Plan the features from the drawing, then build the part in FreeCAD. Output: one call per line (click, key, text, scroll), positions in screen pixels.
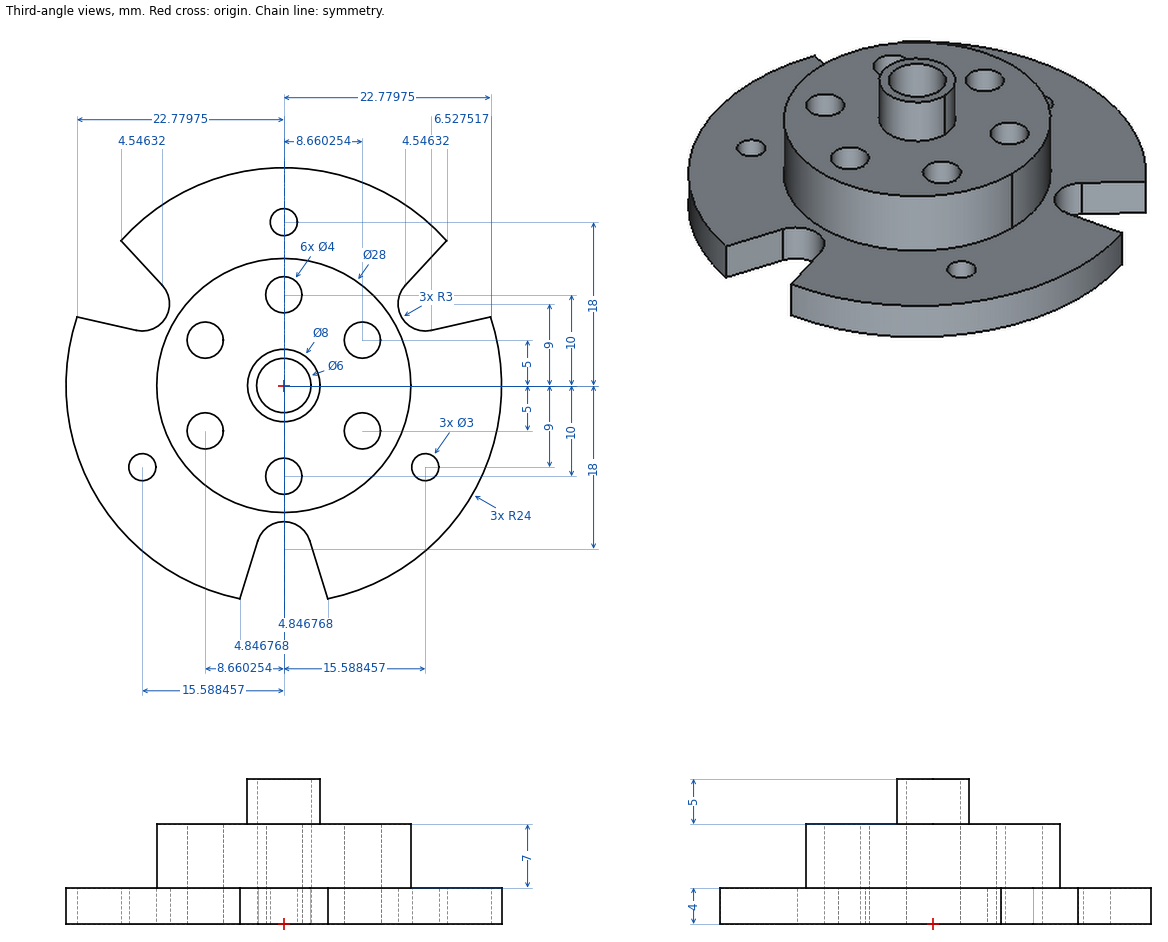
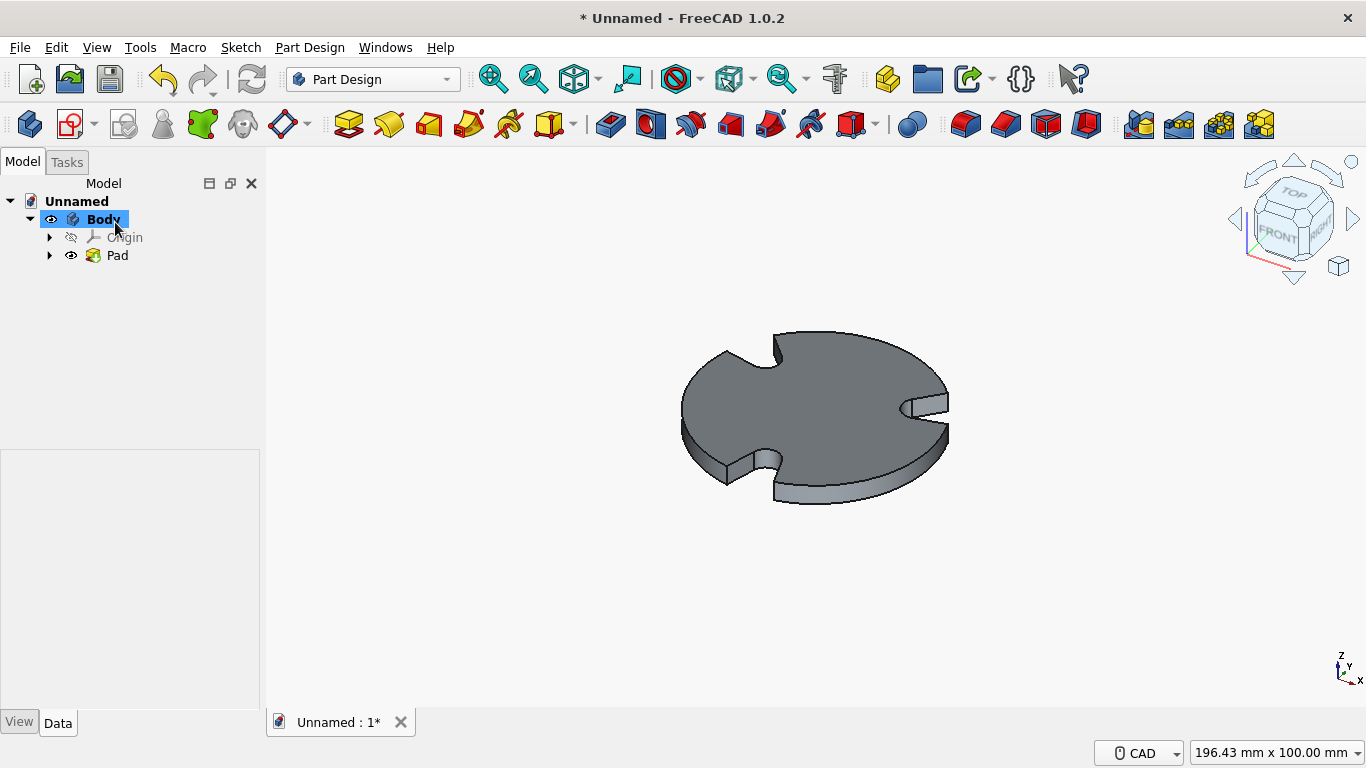
key(v)
key(f)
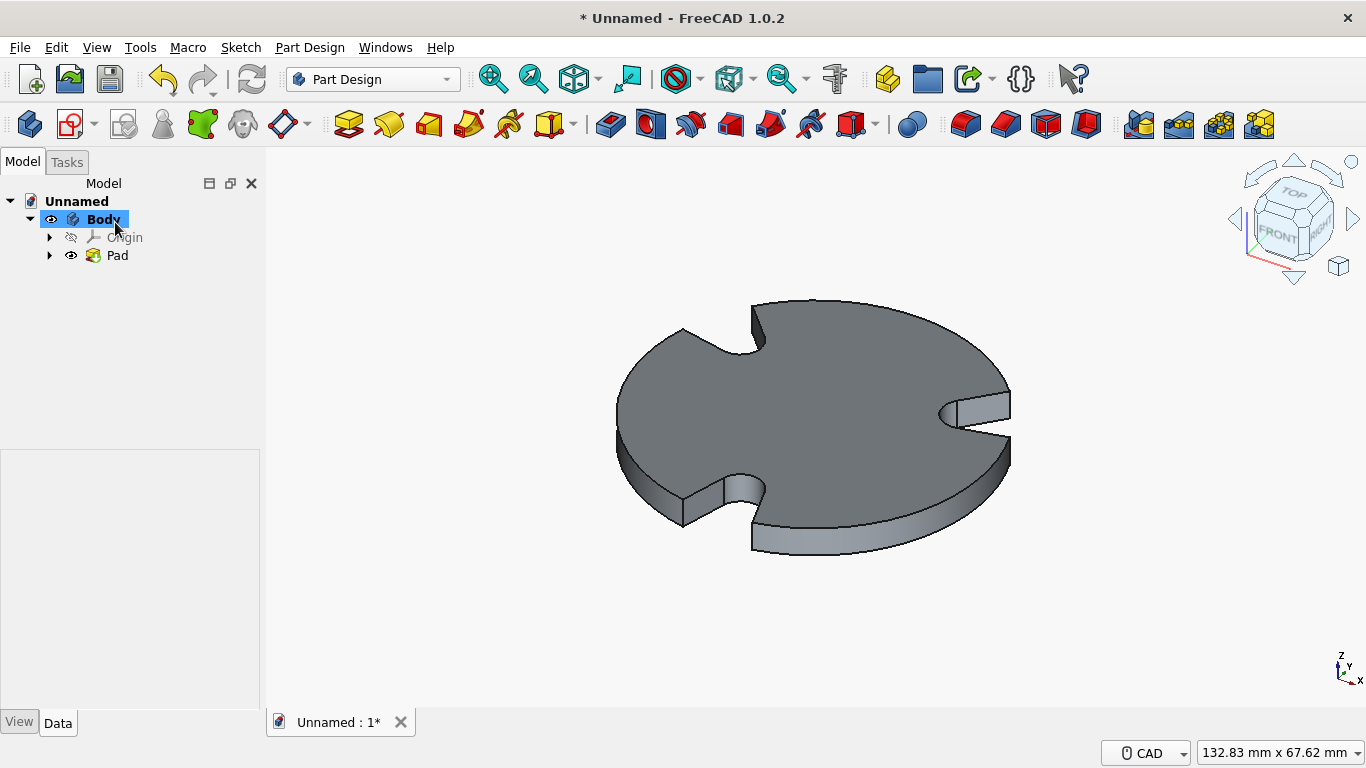
click(816, 412)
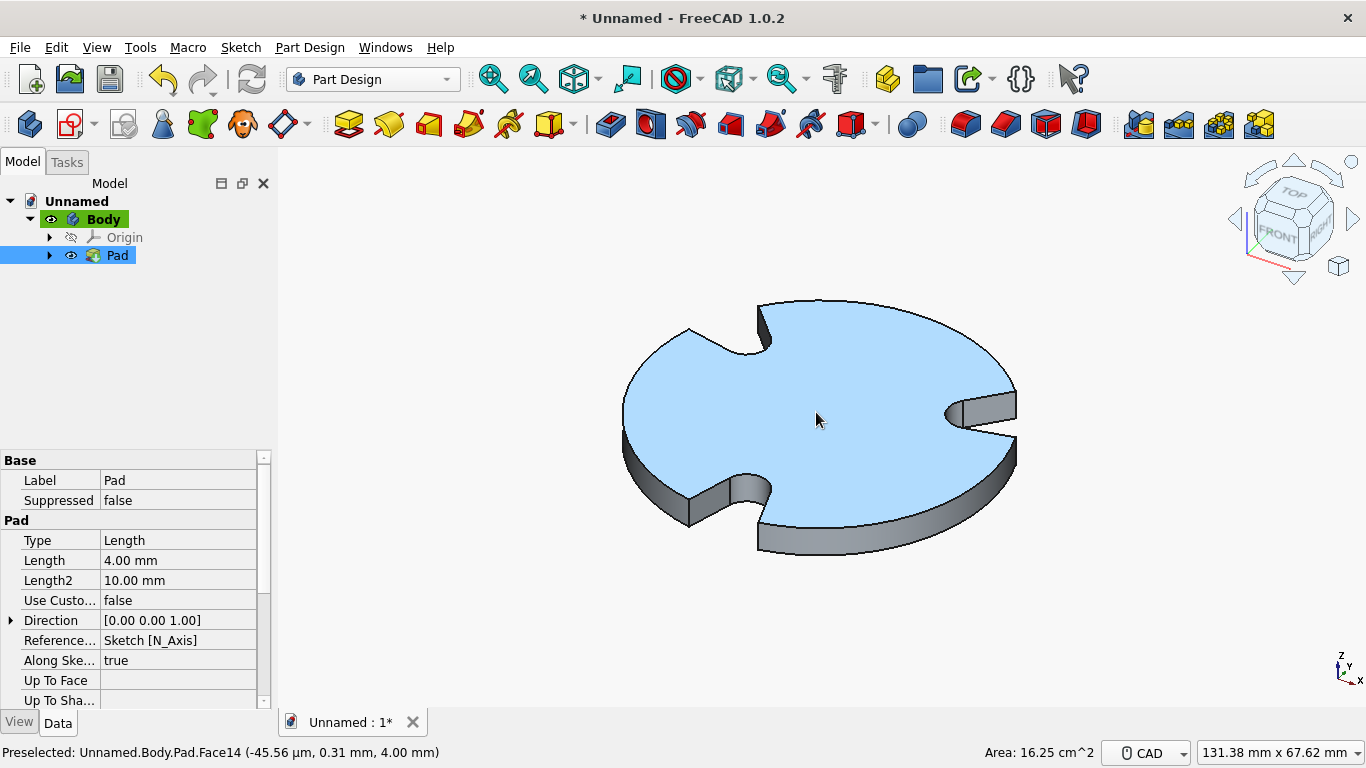
click(70, 124)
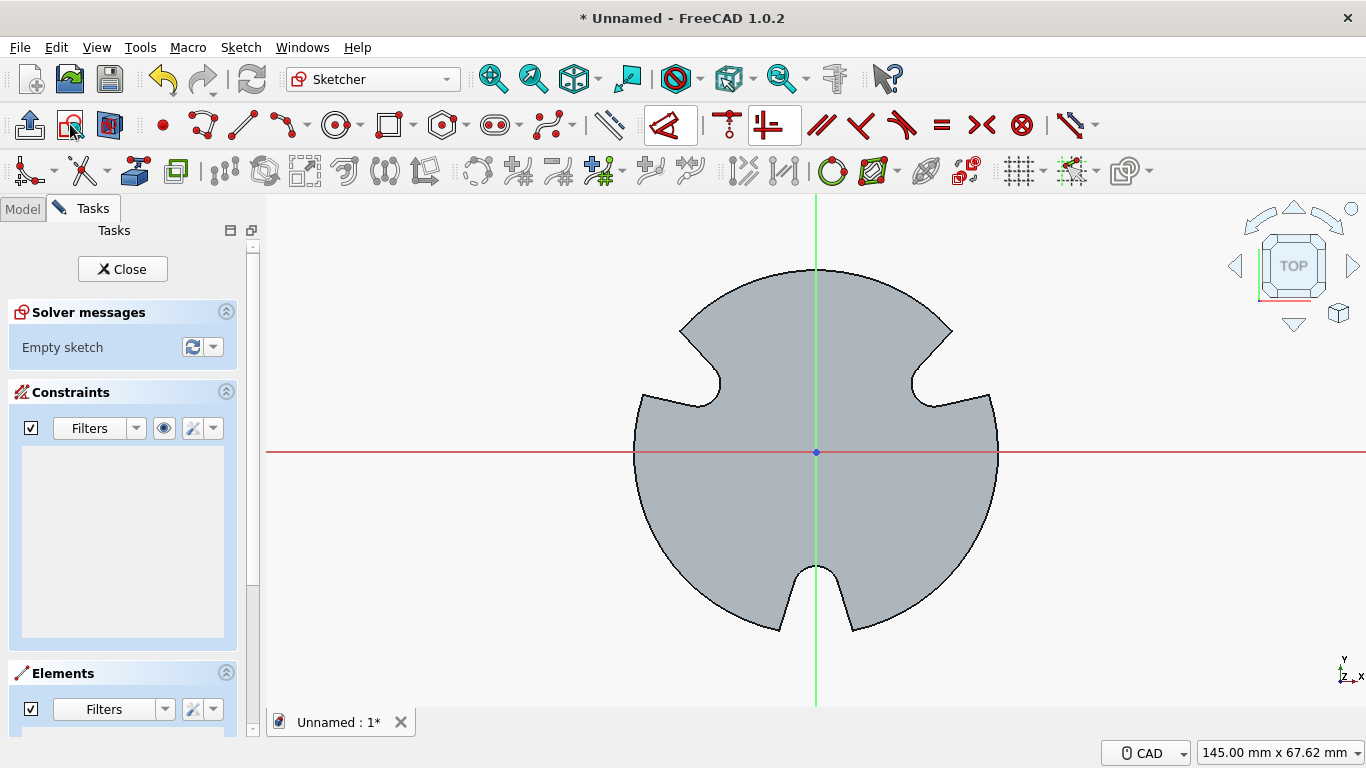
scroll(955, 456, up, 2)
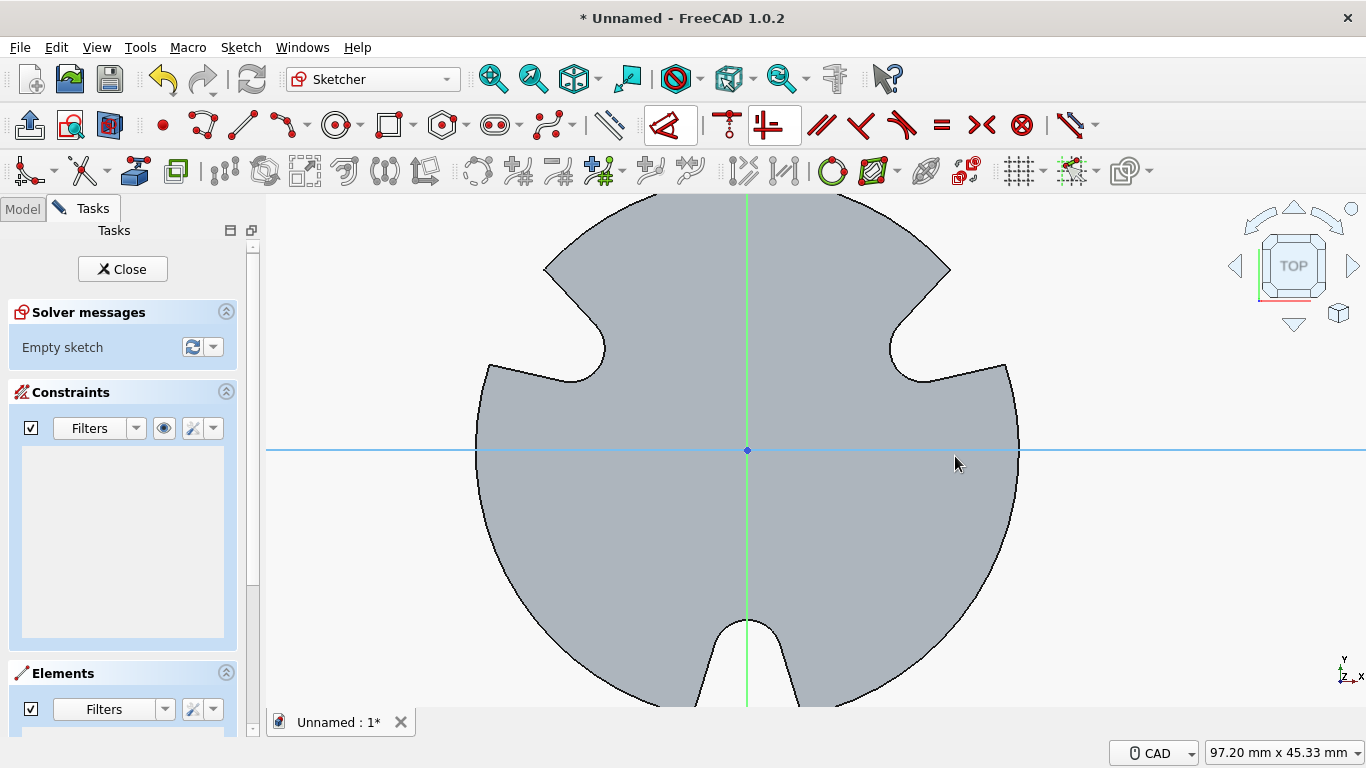
key(g)
key(c)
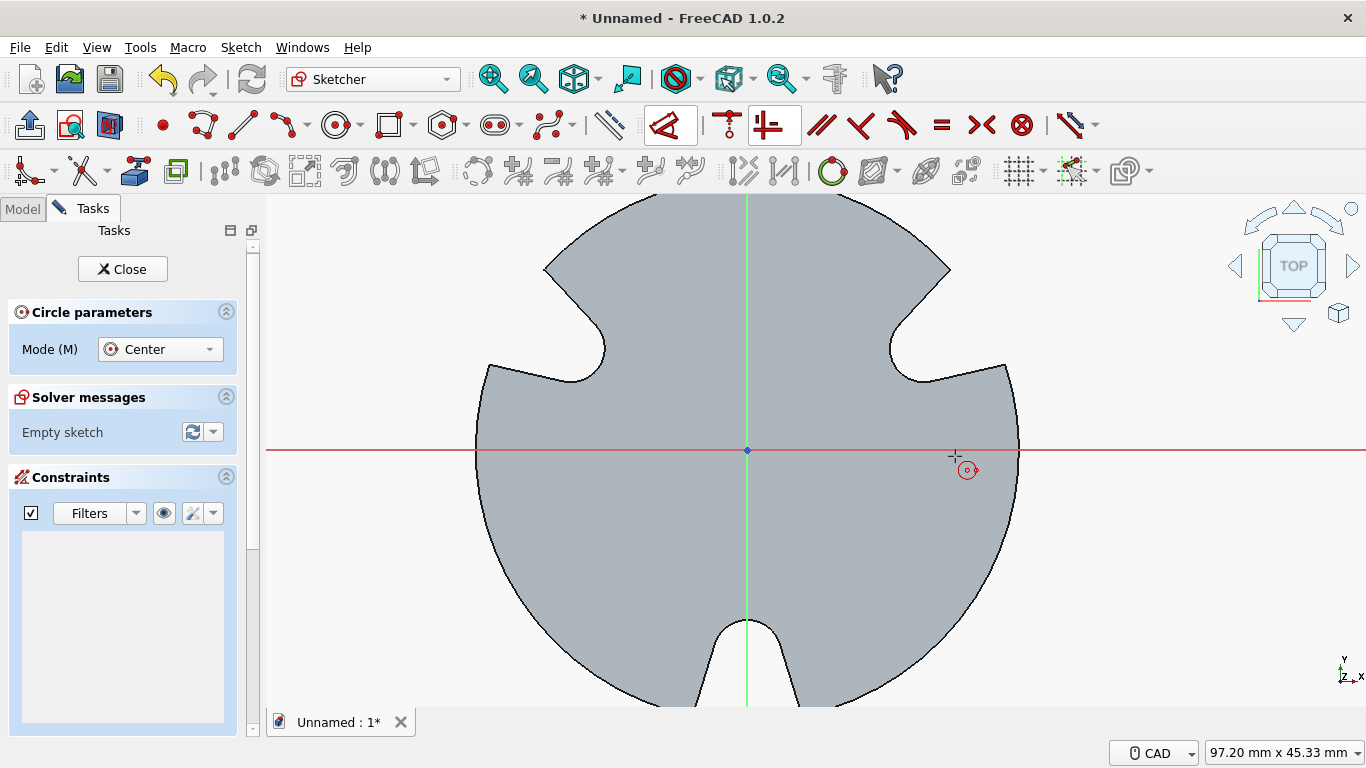
click(747, 450)
click(859, 338)
key(Escape)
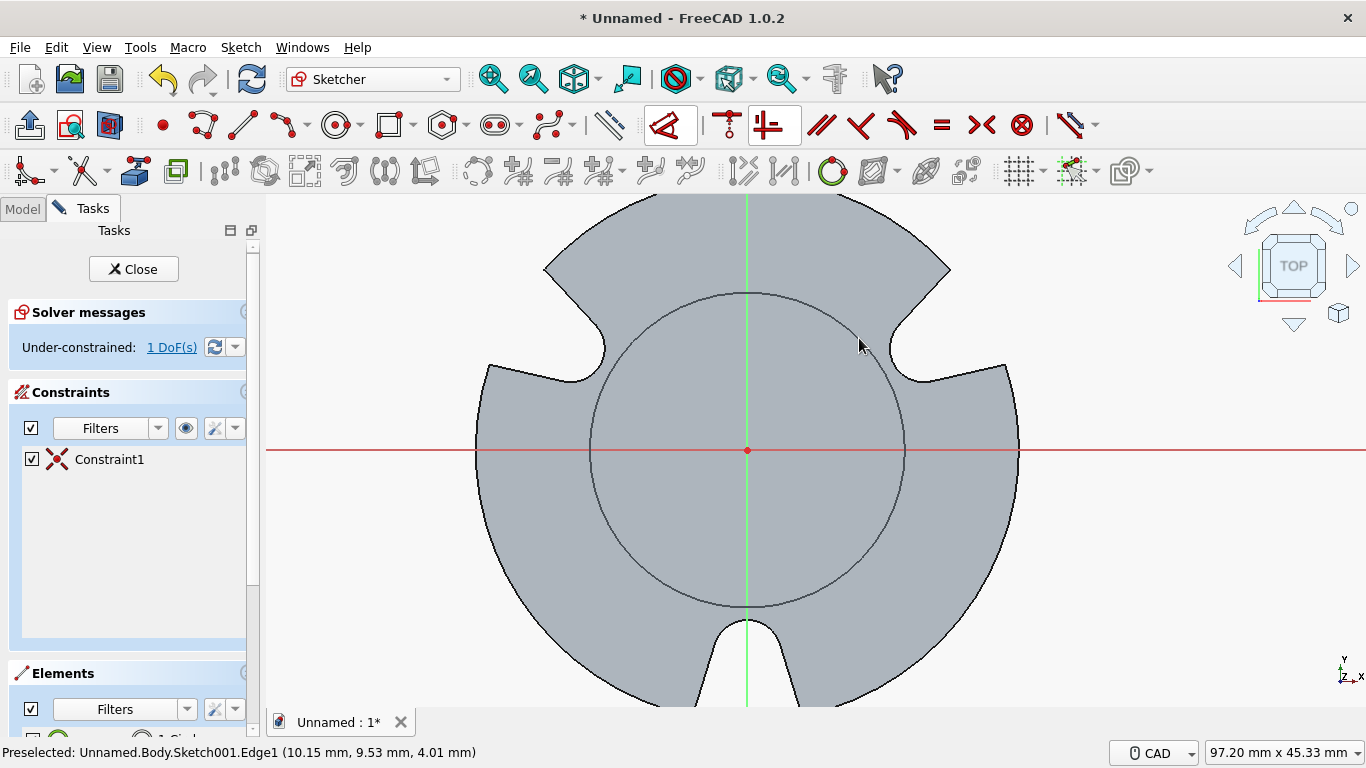
key(d)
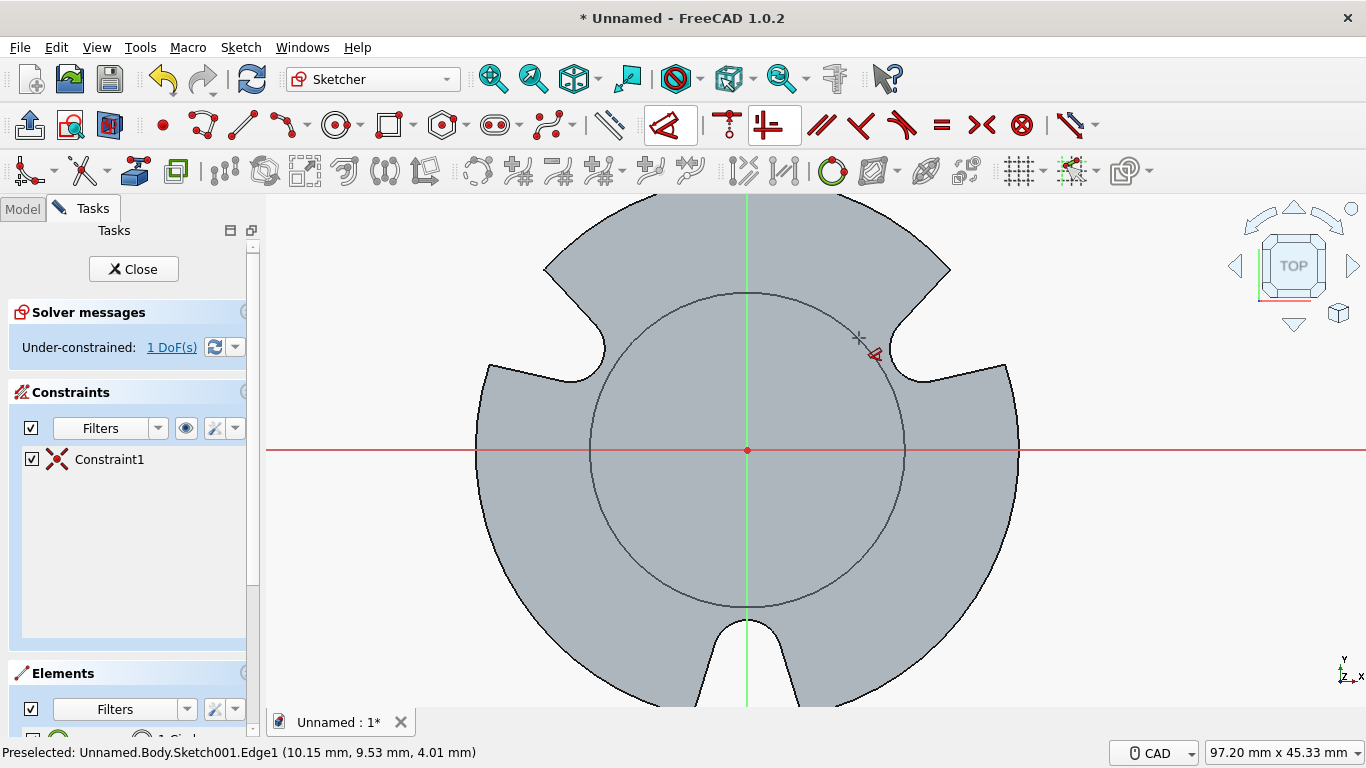
click(858, 338)
click(880, 315)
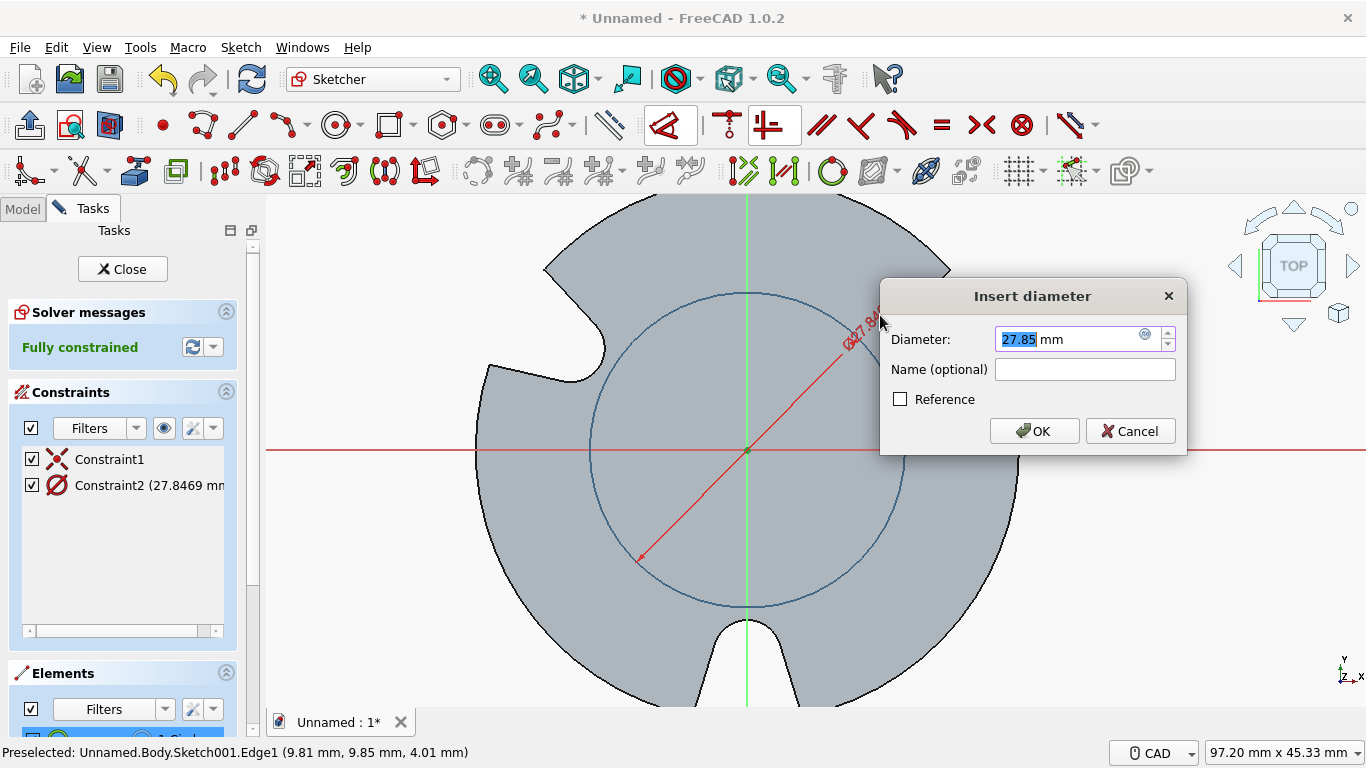
text(28)
key(Return)
key(Escape)